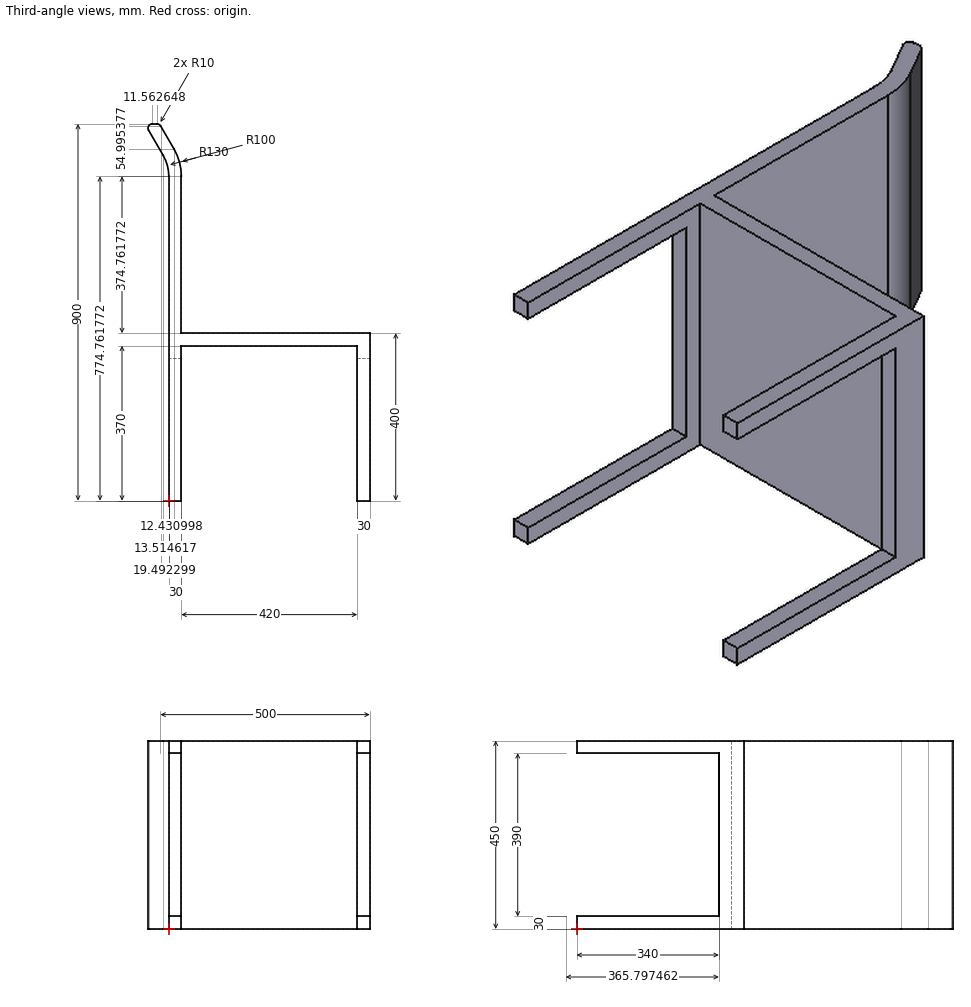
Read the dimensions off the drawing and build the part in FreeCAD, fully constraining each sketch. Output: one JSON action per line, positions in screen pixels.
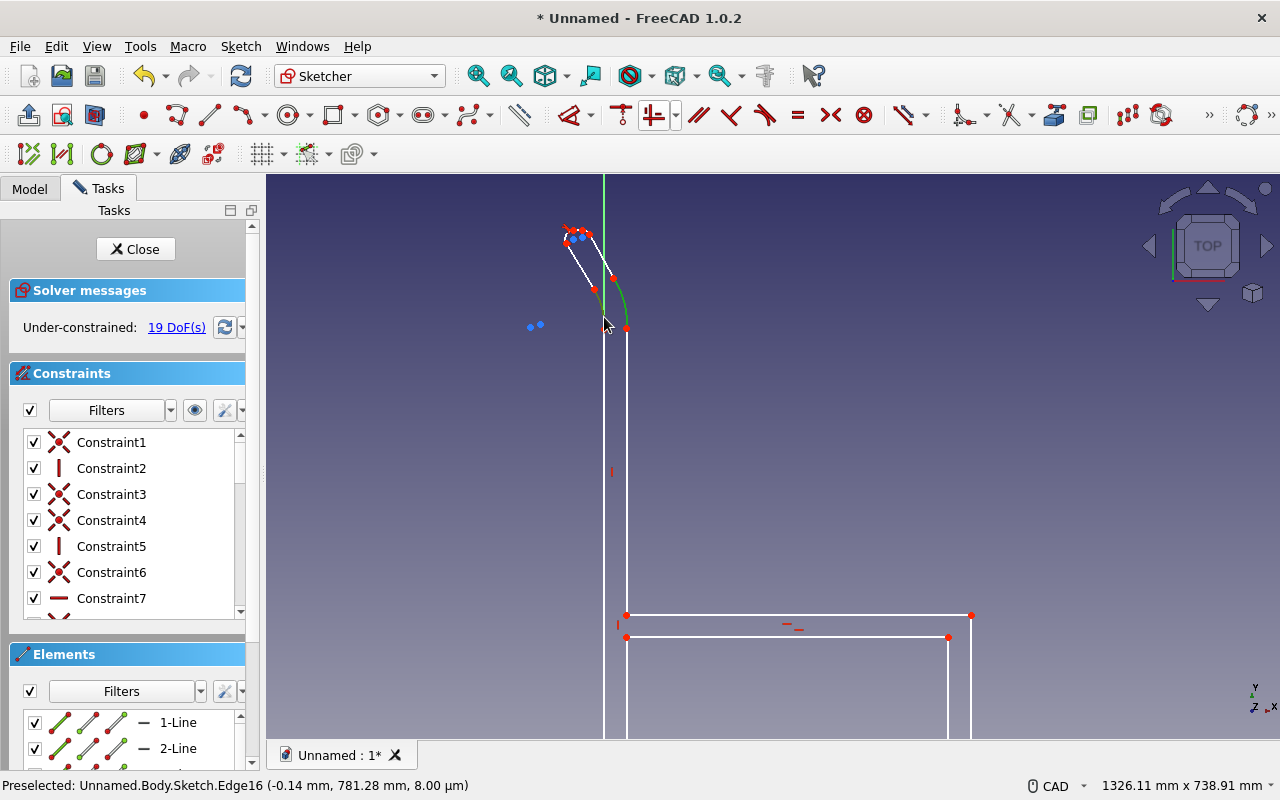
{"action": "left_click", "coordinate": [621, 116]}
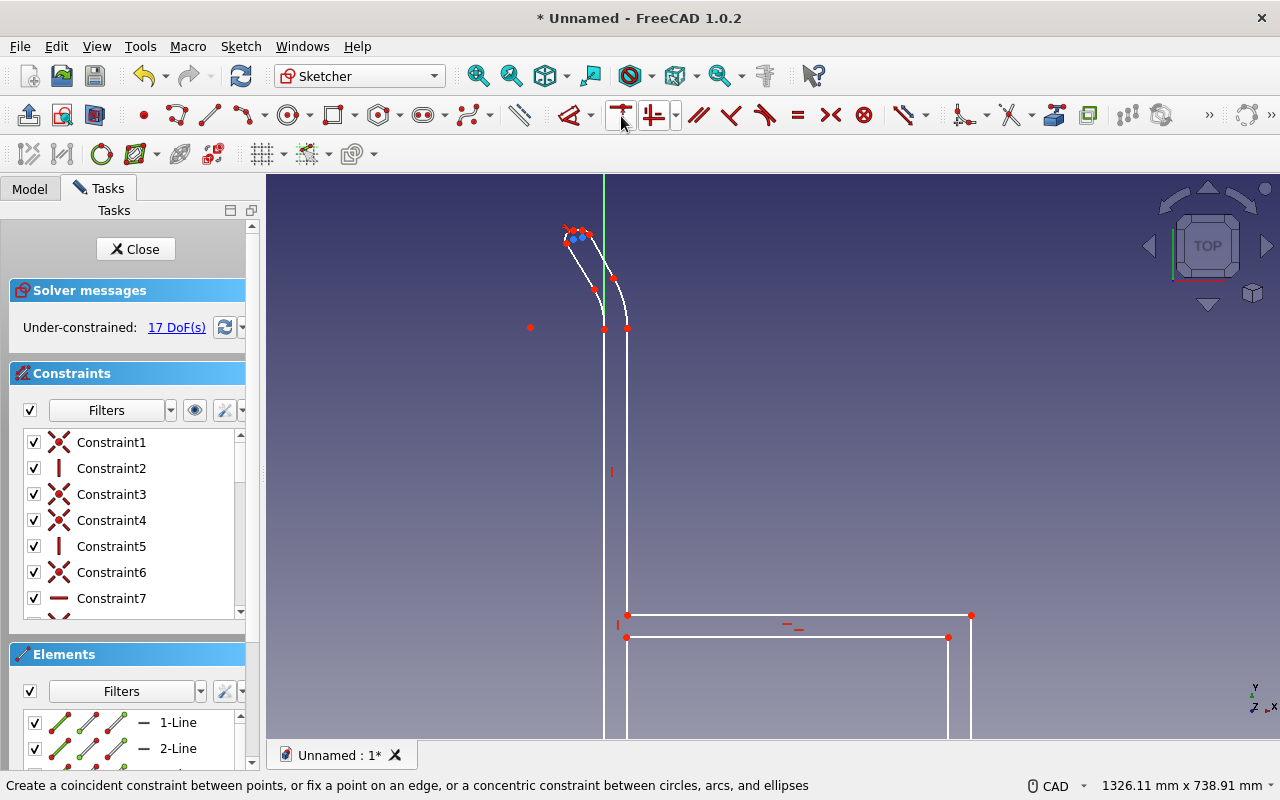
{"action": "scroll", "coordinate": [587, 231], "scroll_direction": "up", "scroll_amount": 7}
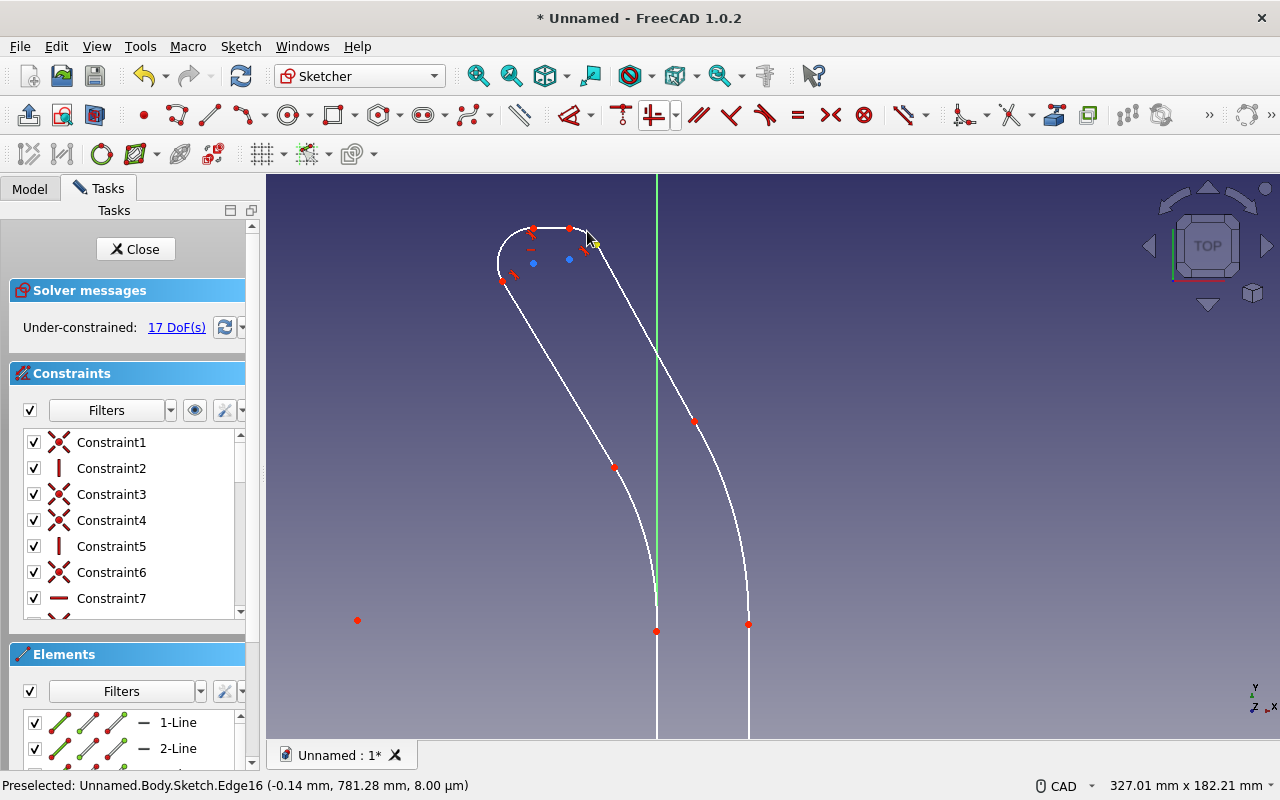
{"action": "left_click", "coordinate": [585, 232]}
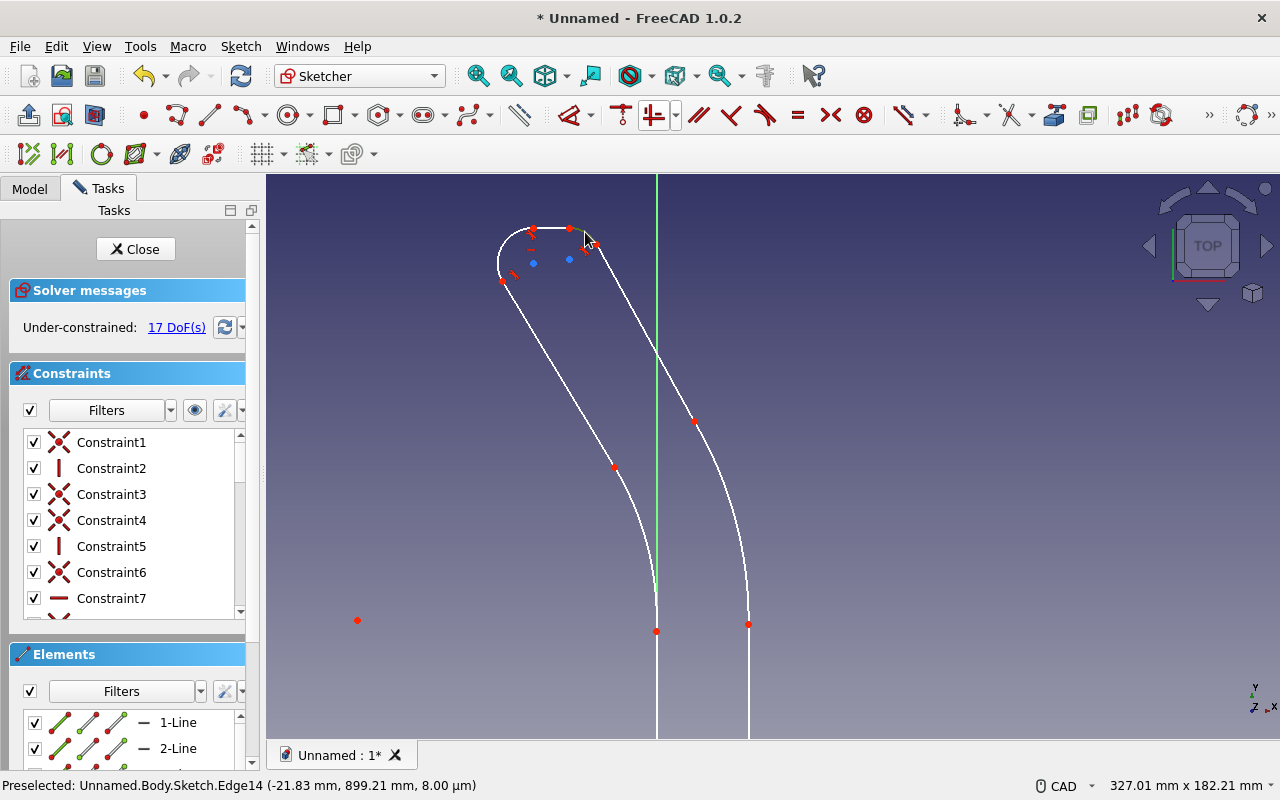
{"action": "left_click", "coordinate": [512, 235]}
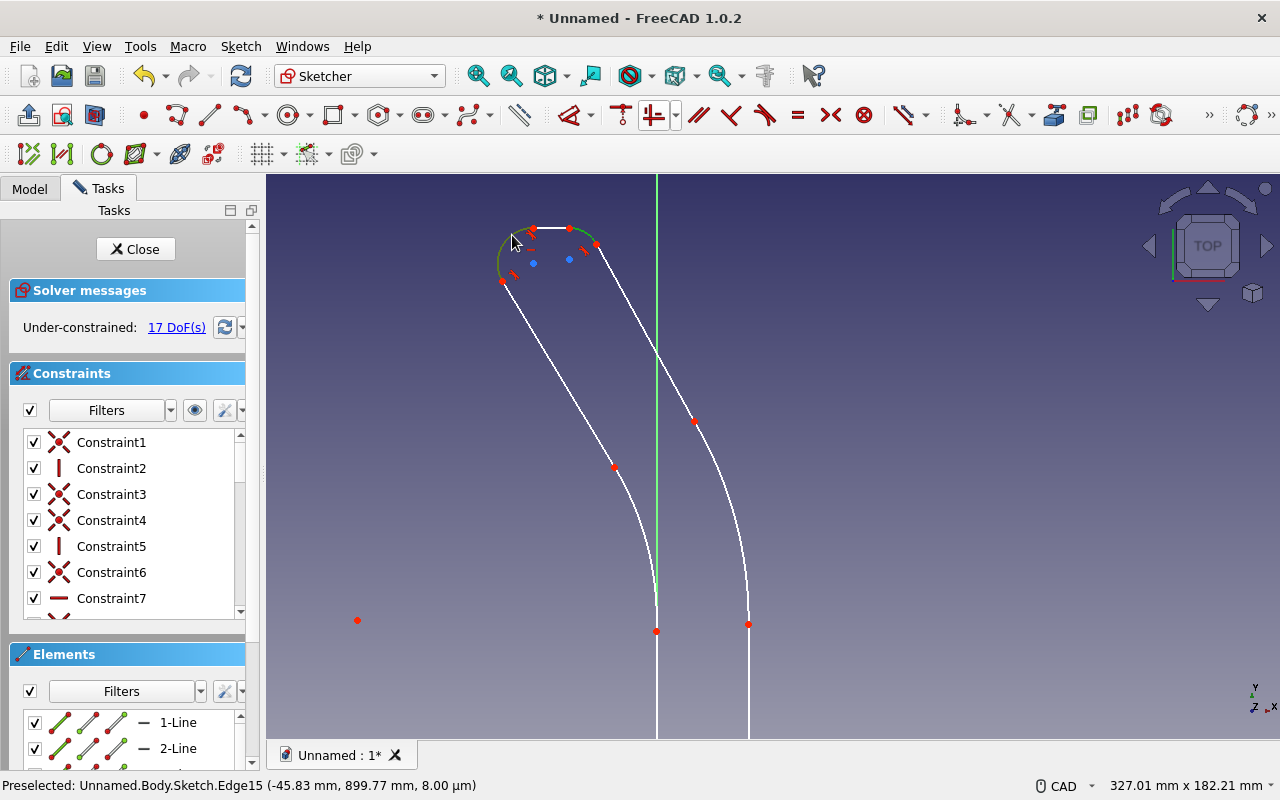
{"action": "left_click", "coordinate": [798, 116]}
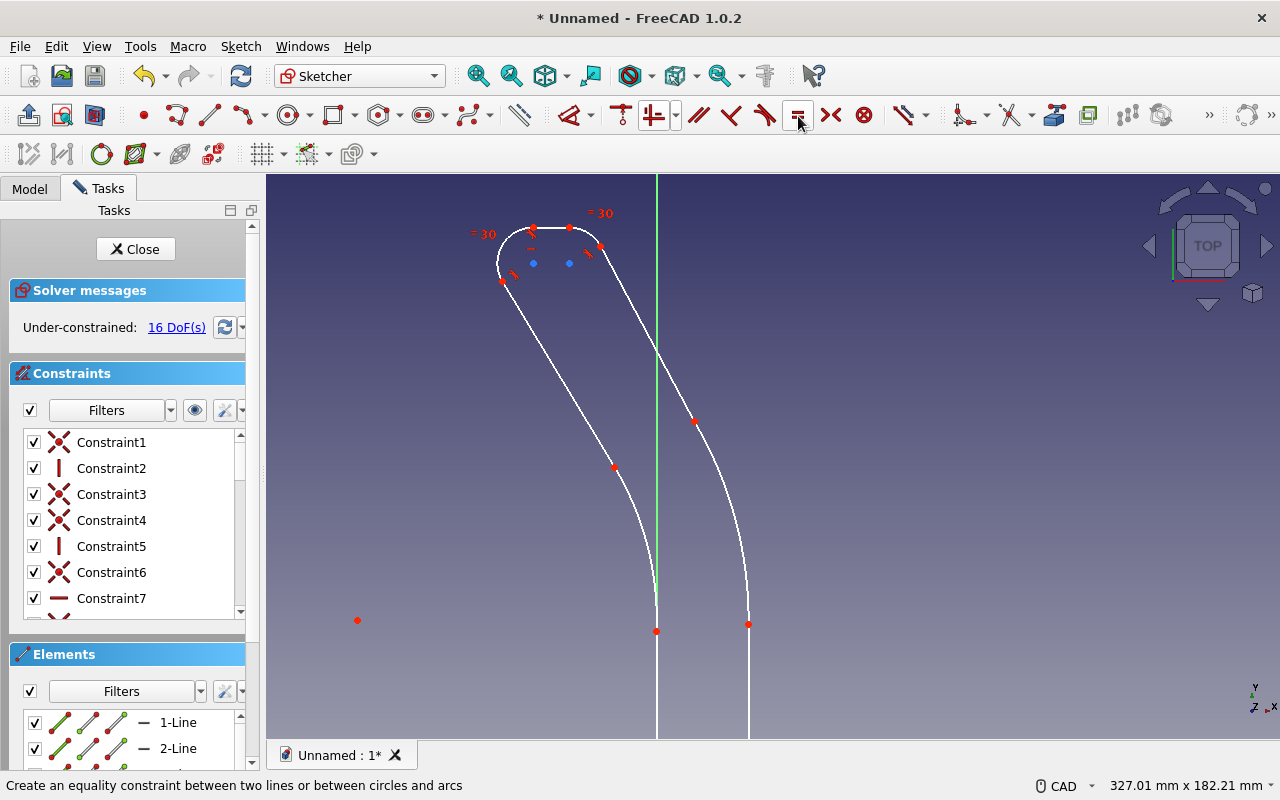
{"action": "scroll", "coordinate": [607, 273], "scroll_direction": "down", "scroll_amount": 10}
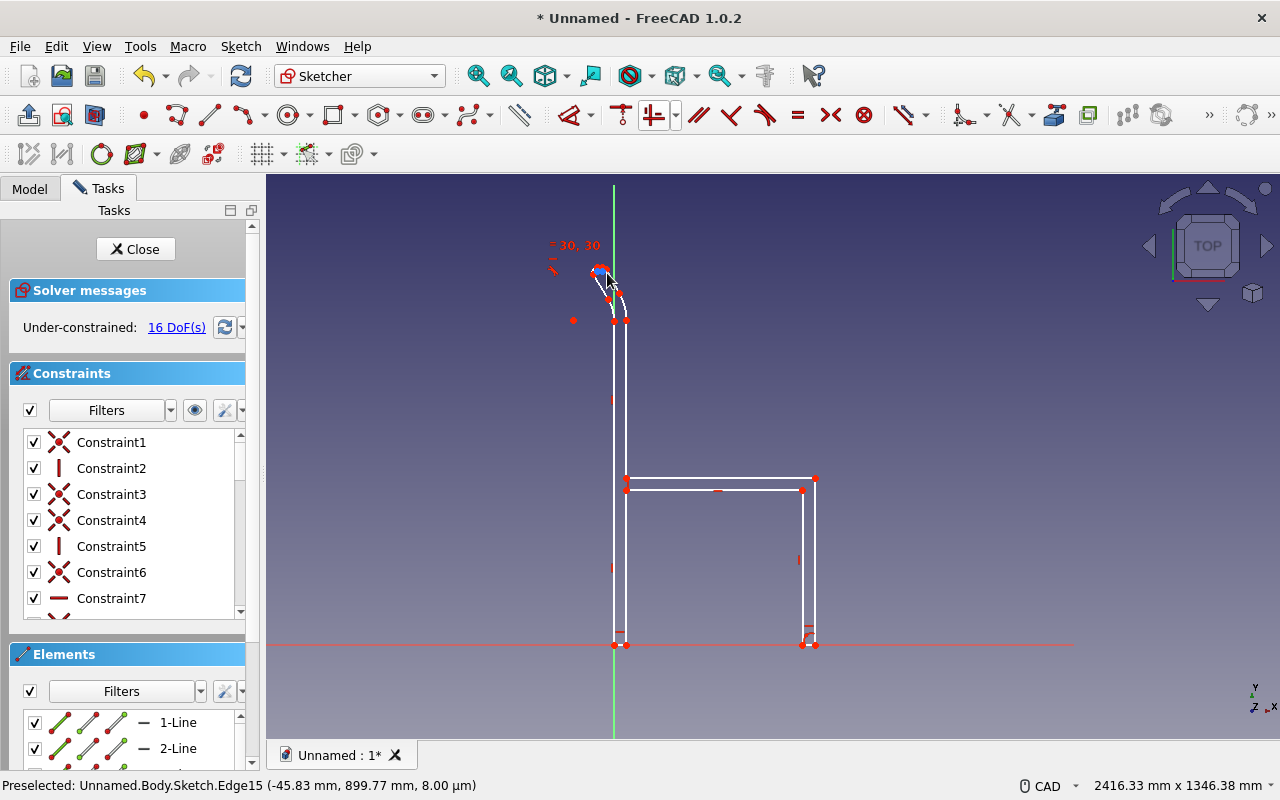
{"action": "scroll", "coordinate": [626, 312], "scroll_direction": "up", "scroll_amount": 3}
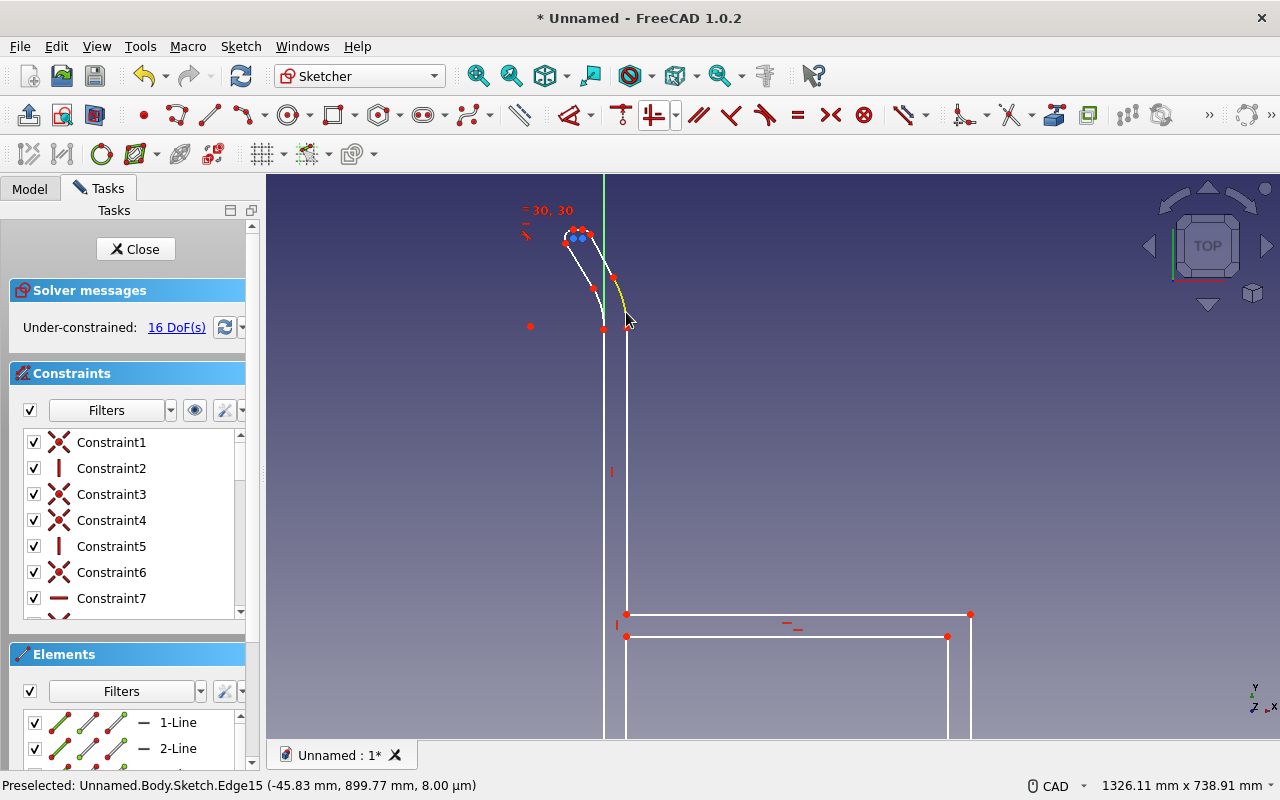
{"action": "left_click", "coordinate": [625, 312]}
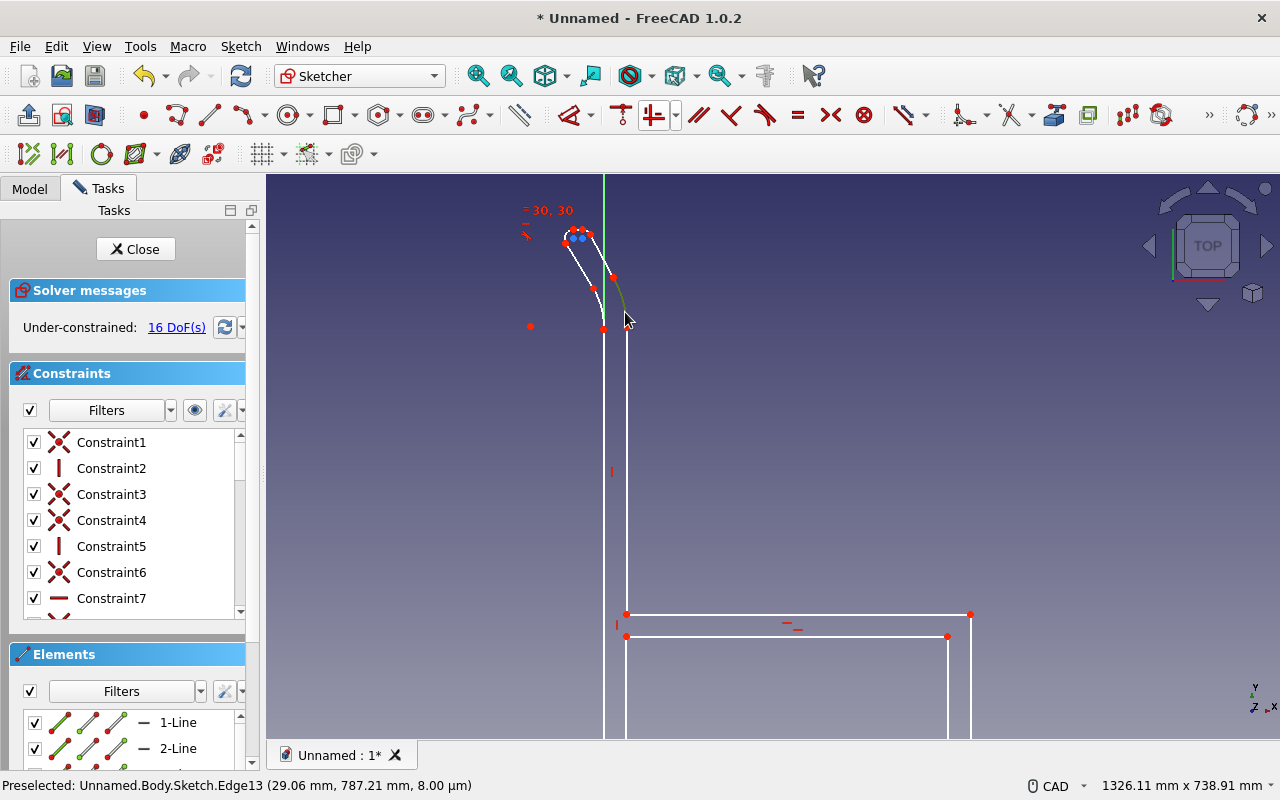
{"action": "key", "text": "k r"}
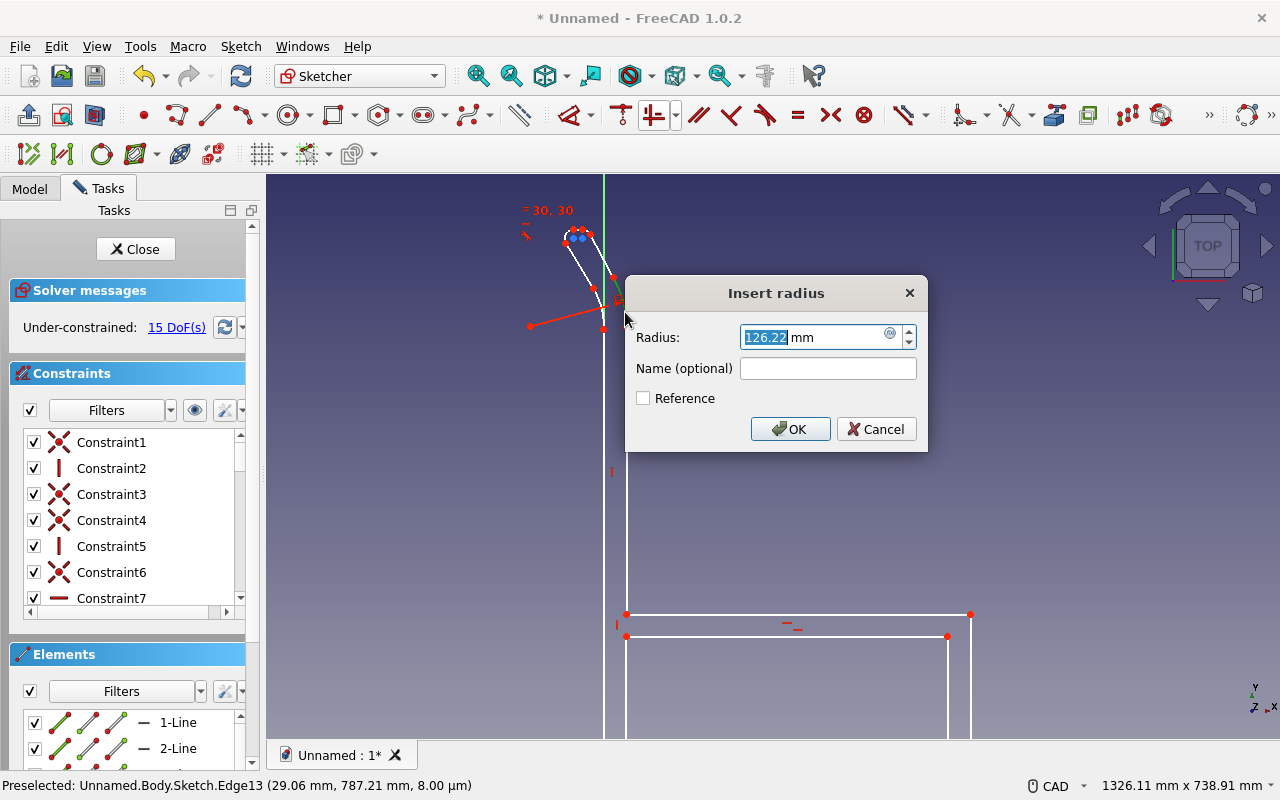
{"action": "type", "text": "130"}
{"action": "key", "text": "Return"}